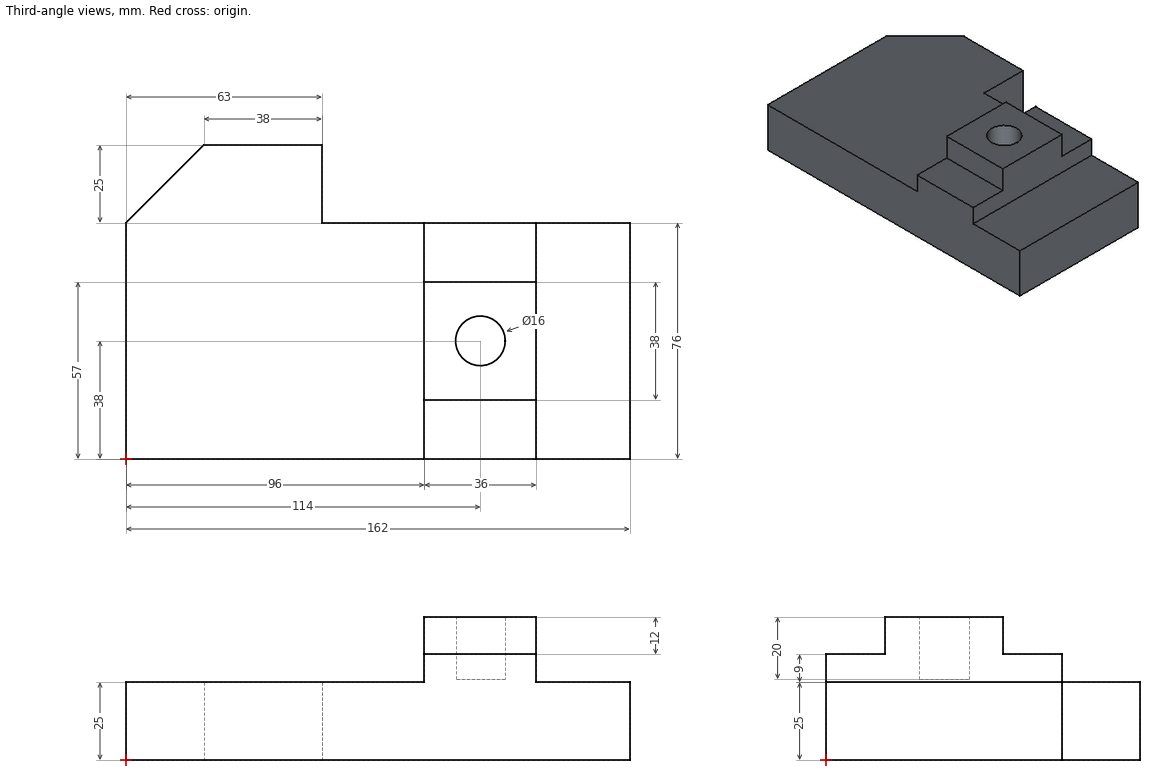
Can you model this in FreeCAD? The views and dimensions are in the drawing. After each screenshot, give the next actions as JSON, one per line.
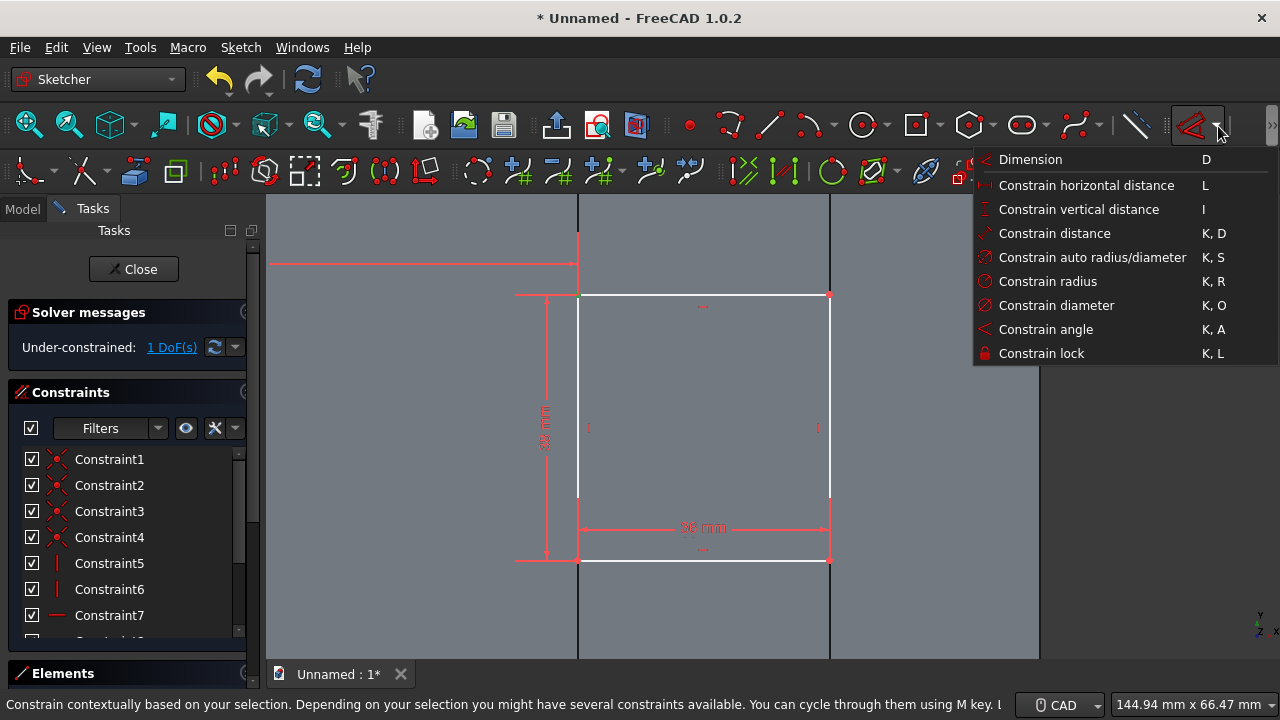
{"action": "left_click", "coordinate": [1126, 209]}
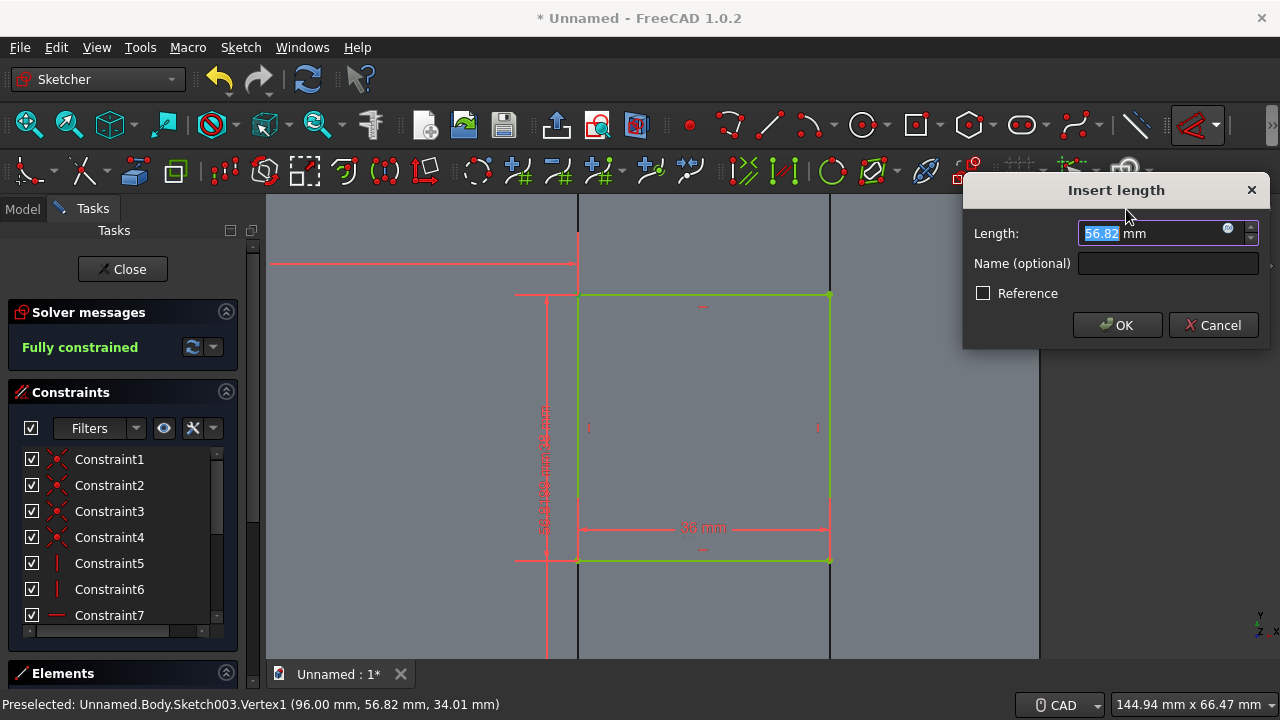
{"action": "type", "text": "57"}
{"action": "key", "text": "Return"}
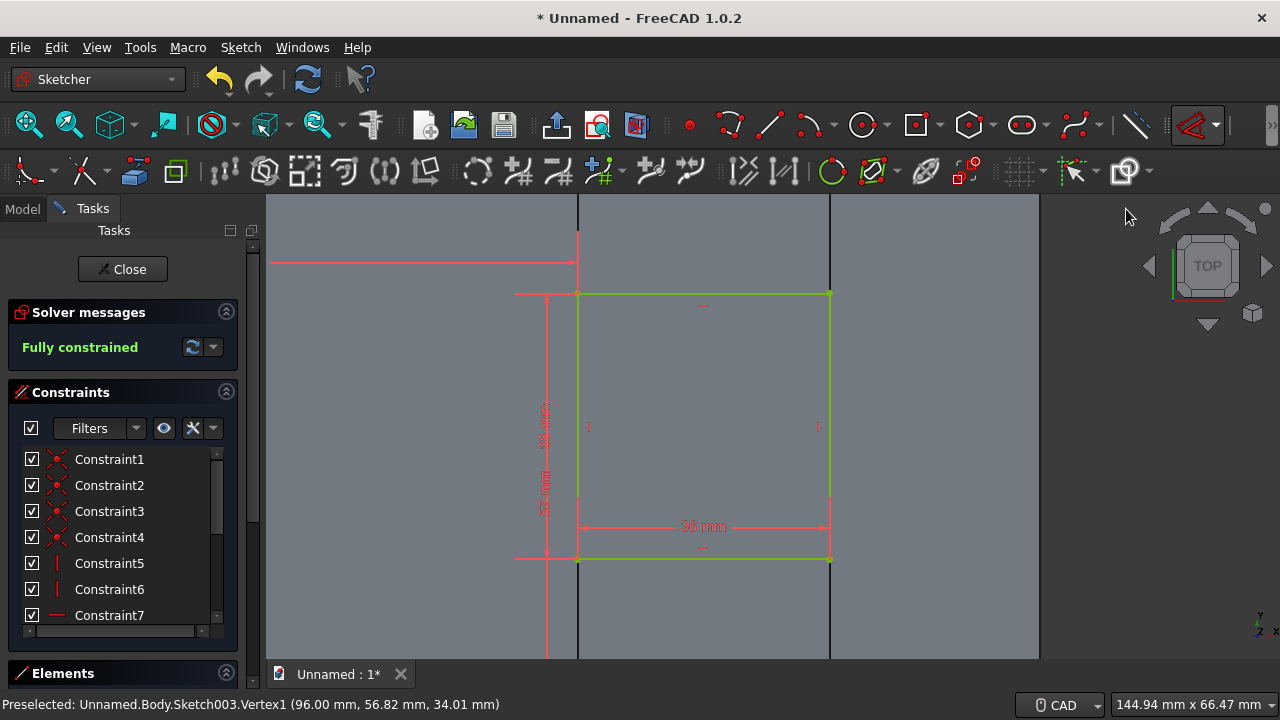
{"action": "left_click", "coordinate": [123, 269]}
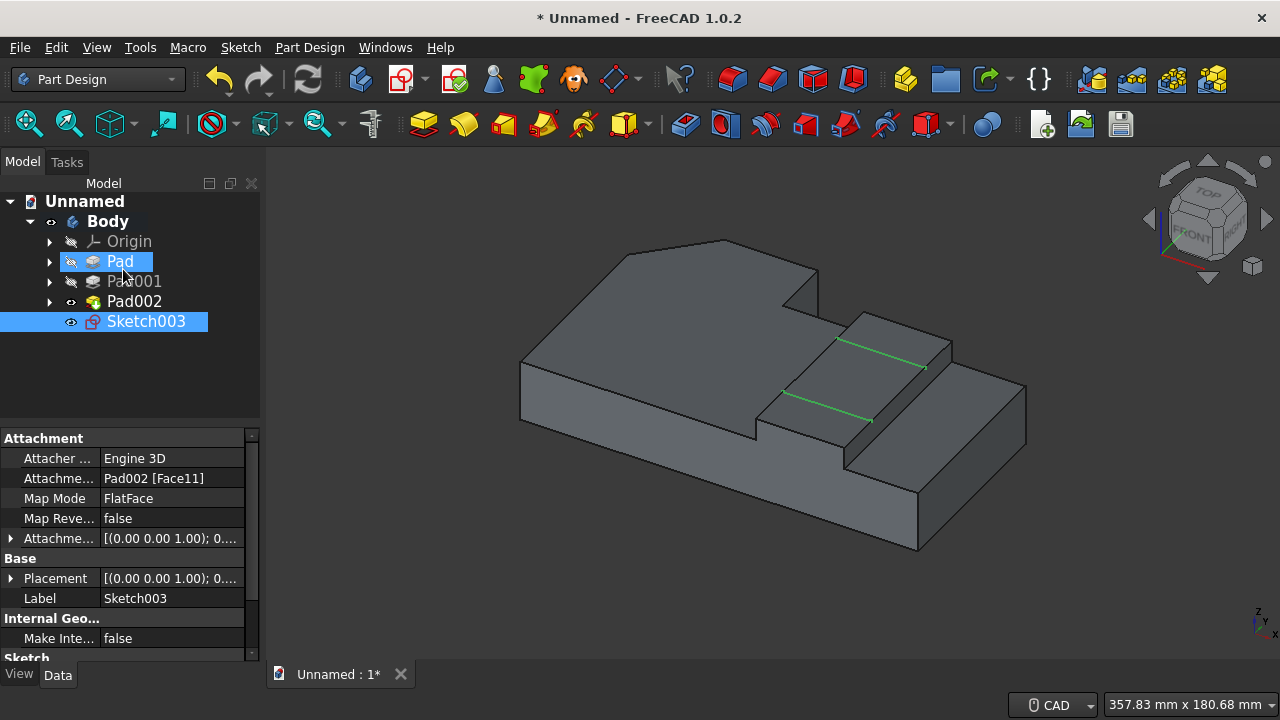
{"action": "left_click", "coordinate": [424, 124]}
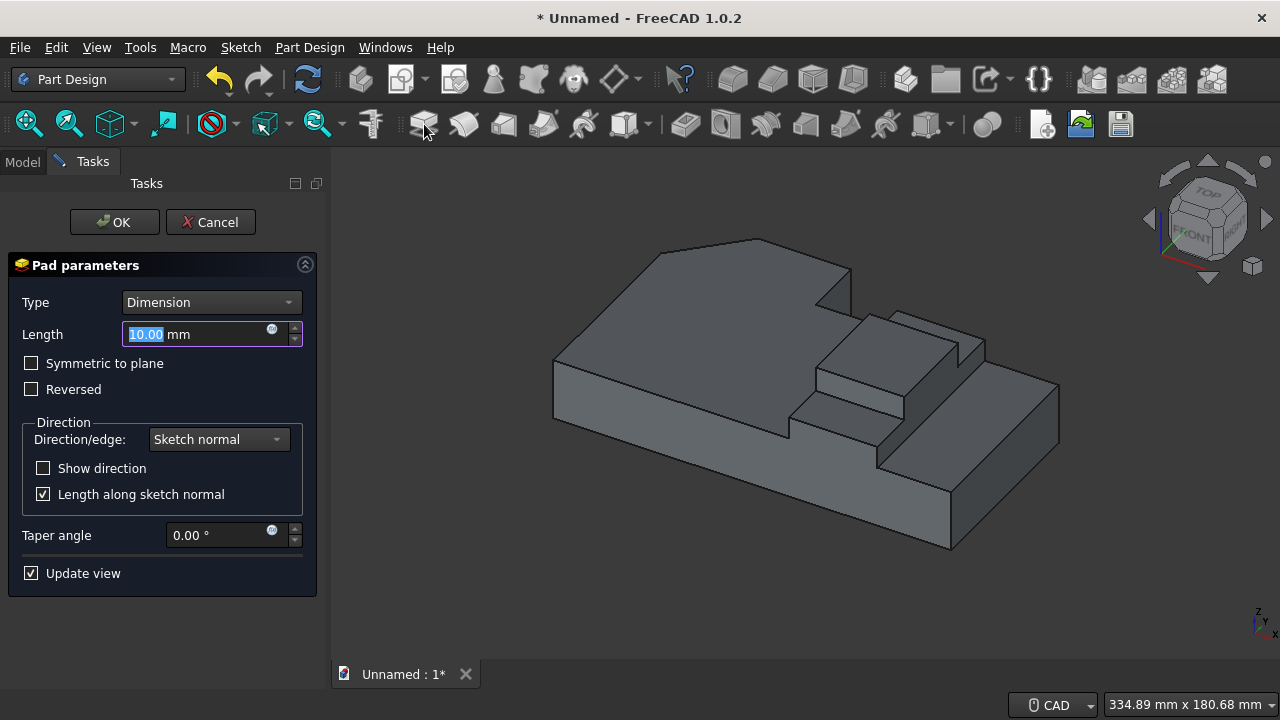
{"action": "type", "text": "12"}
{"action": "key", "text": "Tab"}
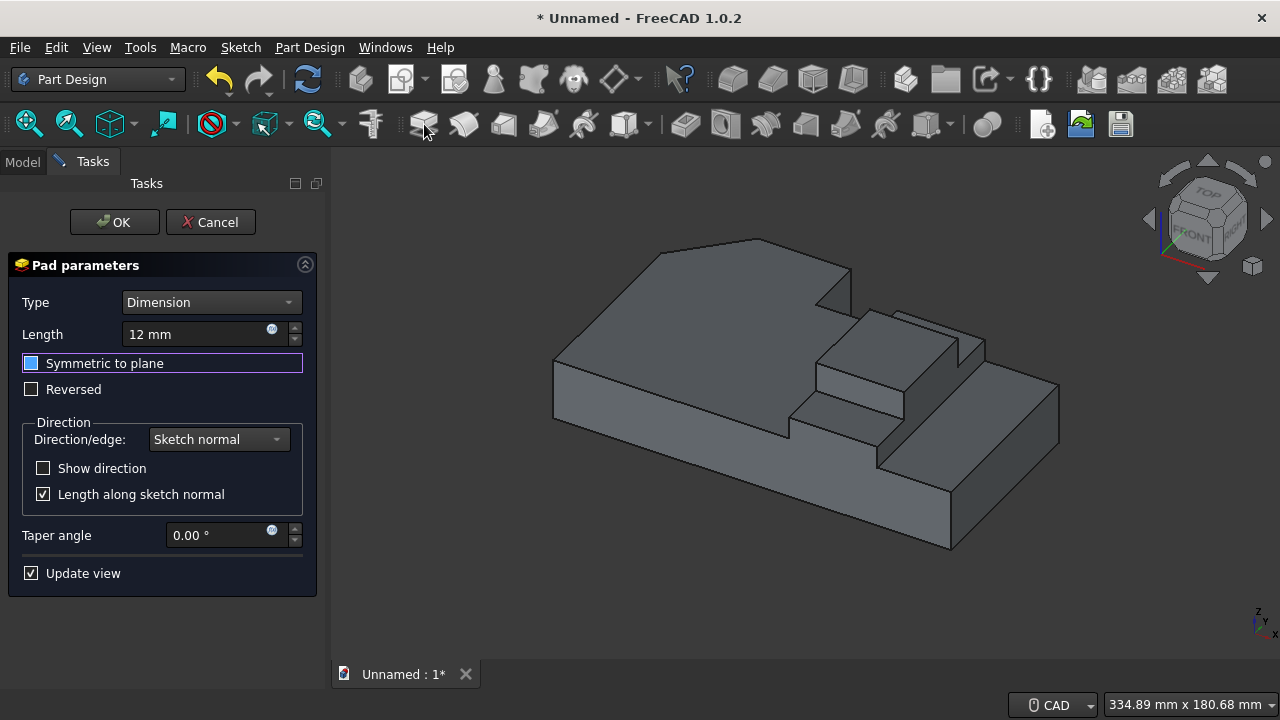
{"action": "left_click", "coordinate": [115, 222]}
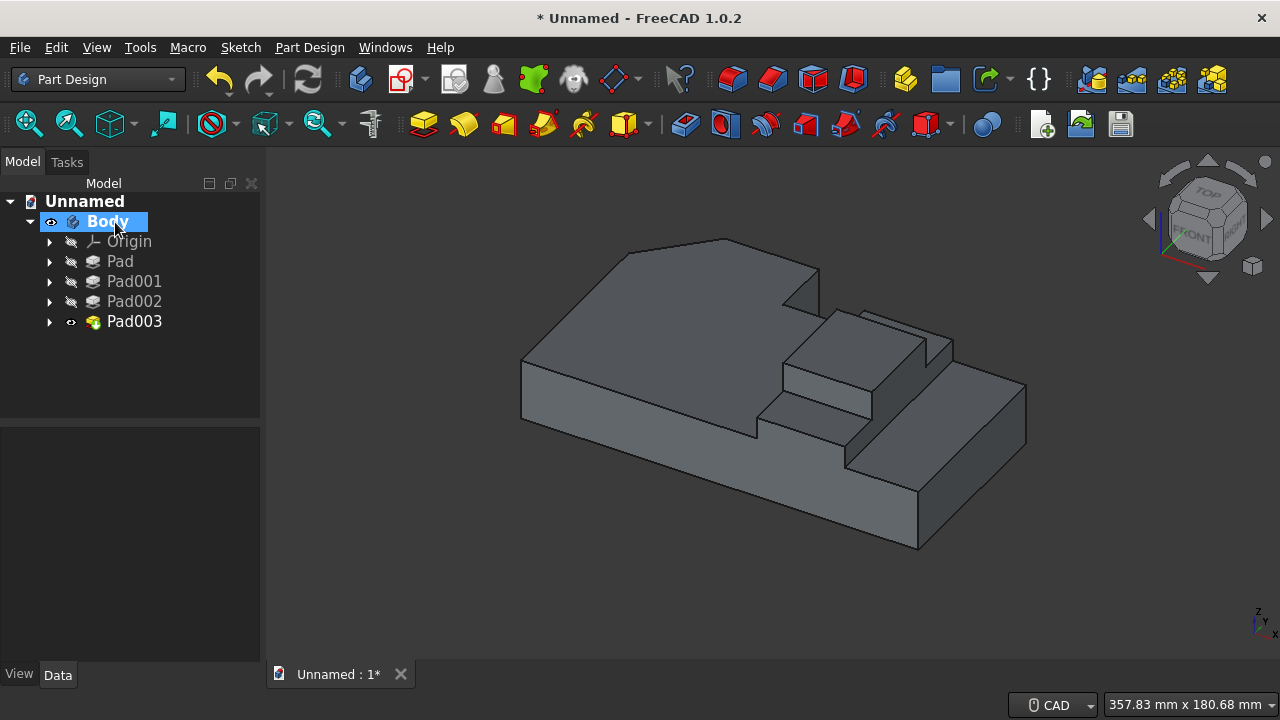
{"action": "left_click", "coordinate": [855, 350]}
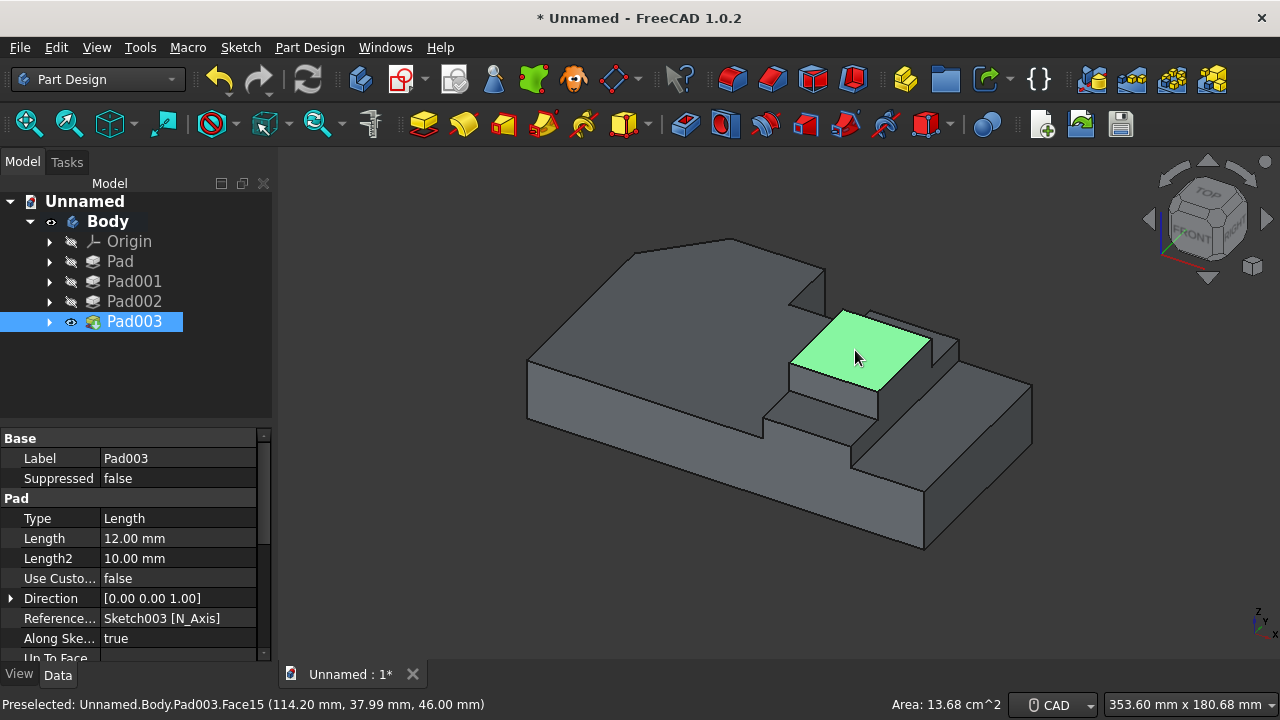
{"action": "left_click", "coordinate": [402, 80]}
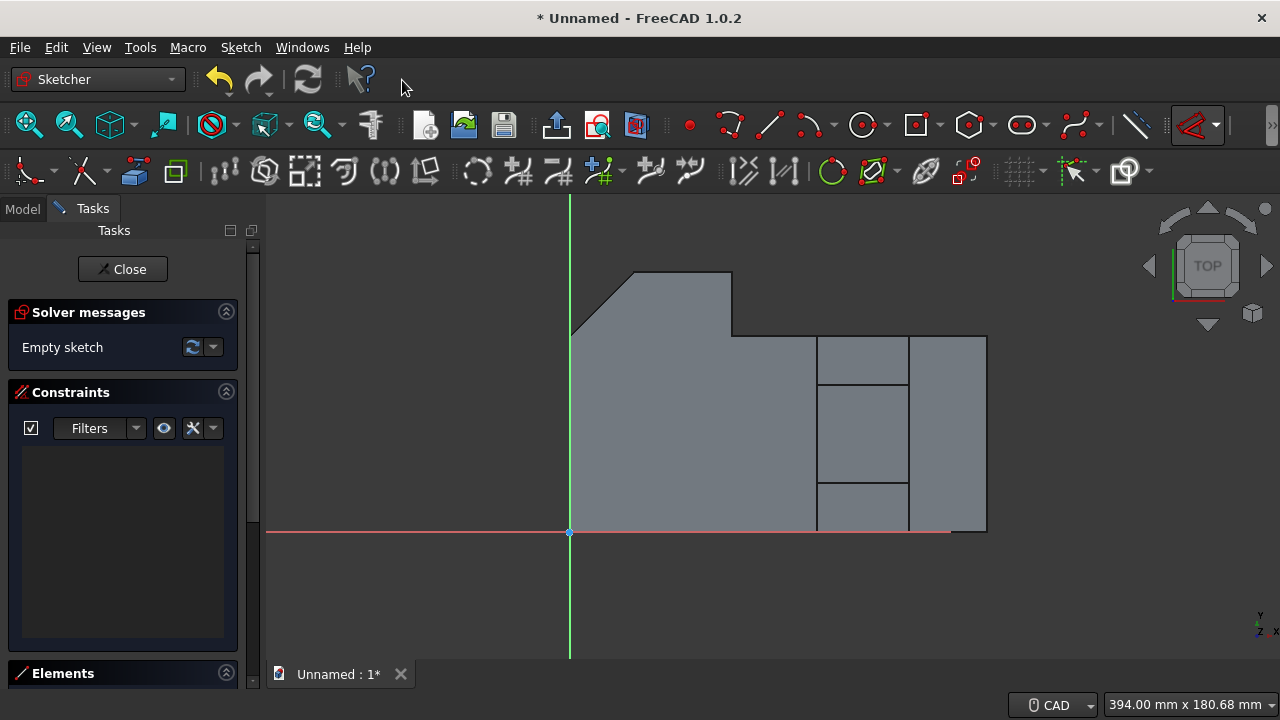
{"action": "scroll", "coordinate": [888, 435], "scroll_direction": "up", "scroll_amount": 10}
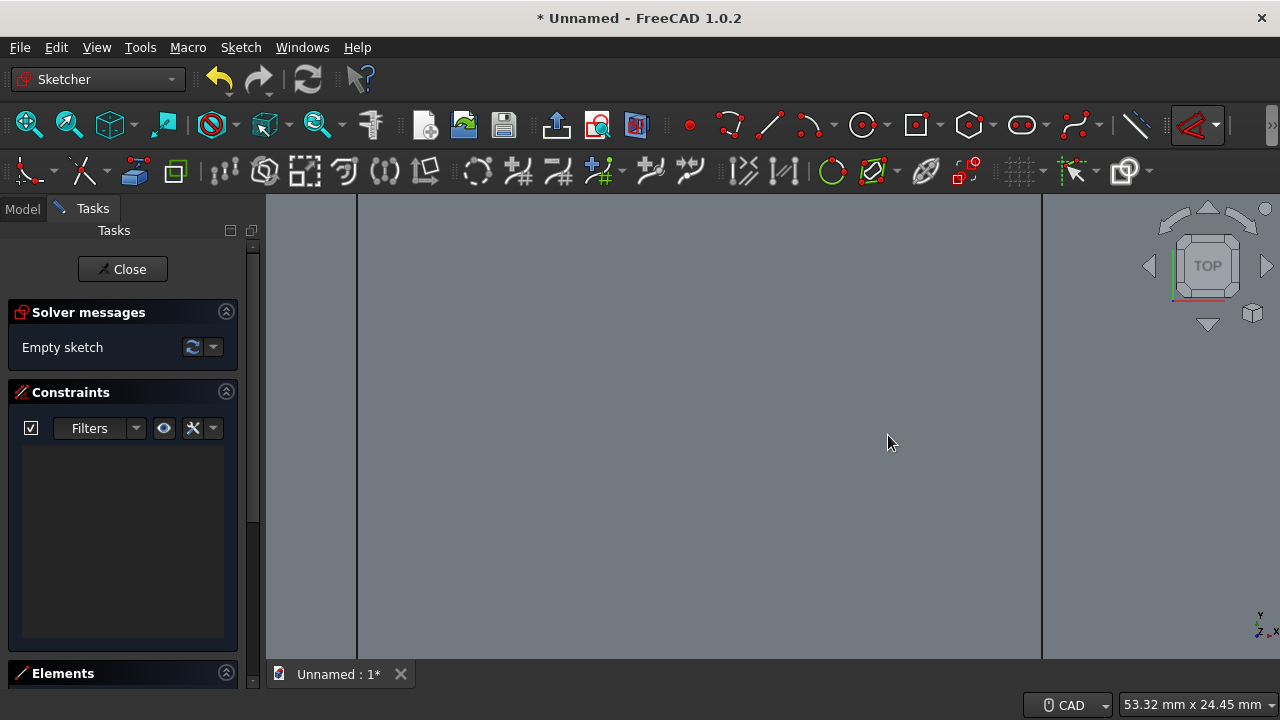
{"action": "left_click", "coordinate": [864, 126]}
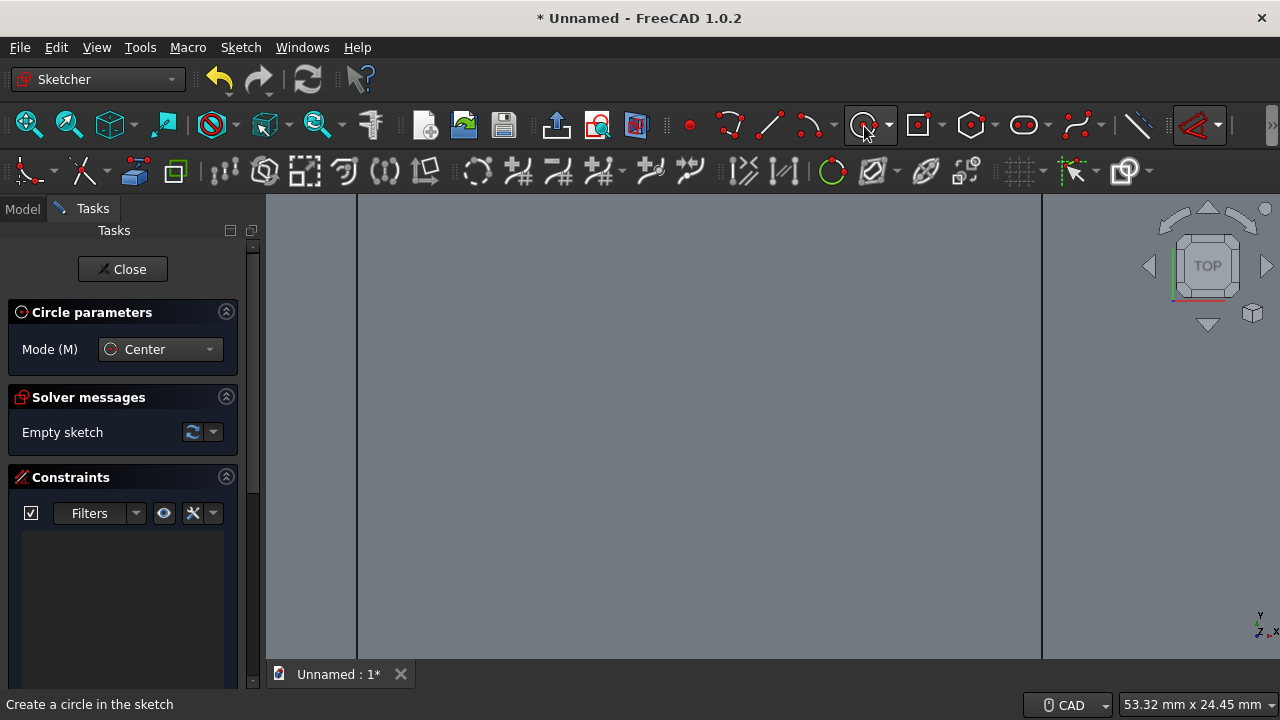
{"action": "left_click", "coordinate": [699, 426]}
{"action": "left_click", "coordinate": [807, 319]}
{"action": "key", "text": "Escape"}